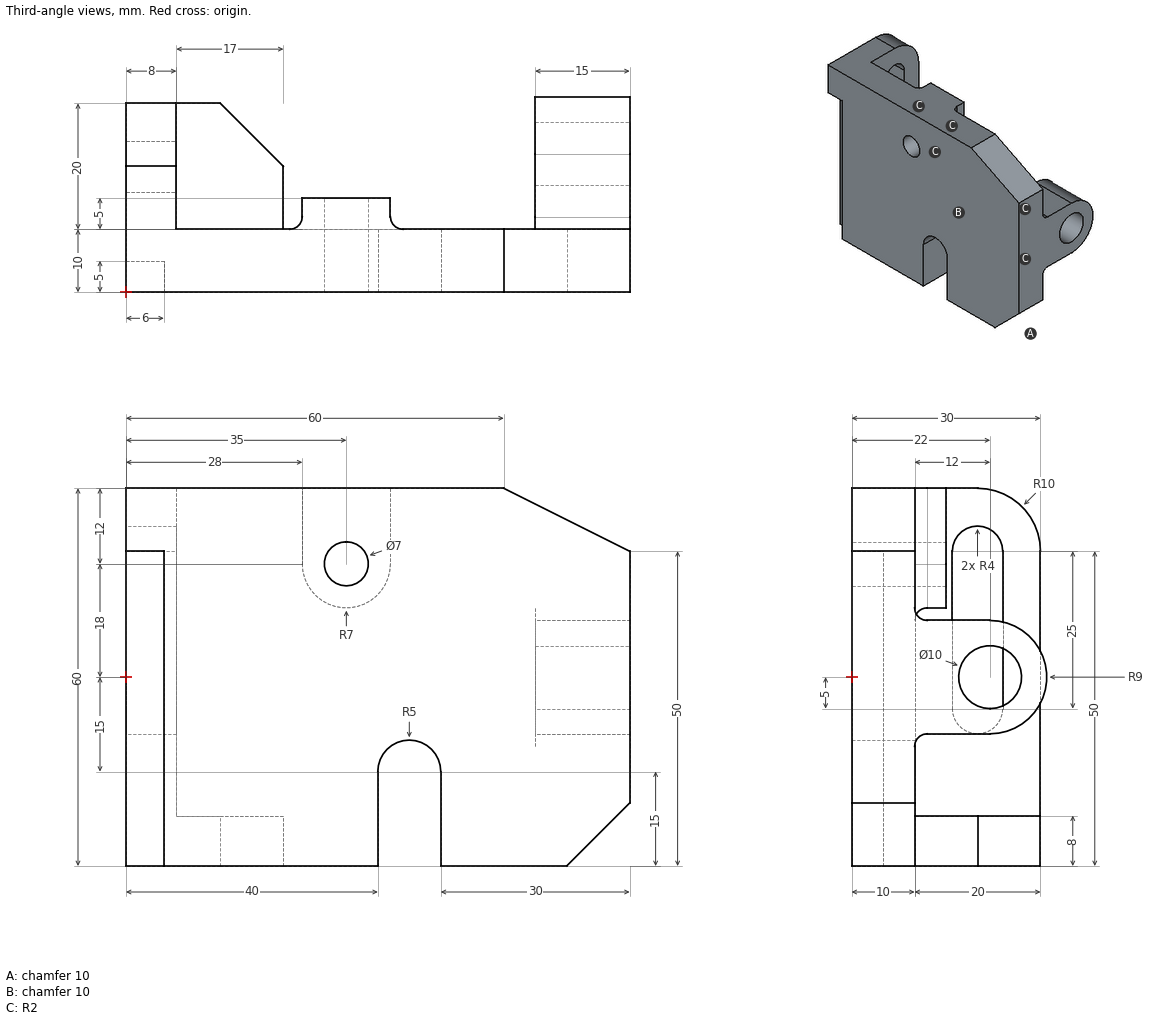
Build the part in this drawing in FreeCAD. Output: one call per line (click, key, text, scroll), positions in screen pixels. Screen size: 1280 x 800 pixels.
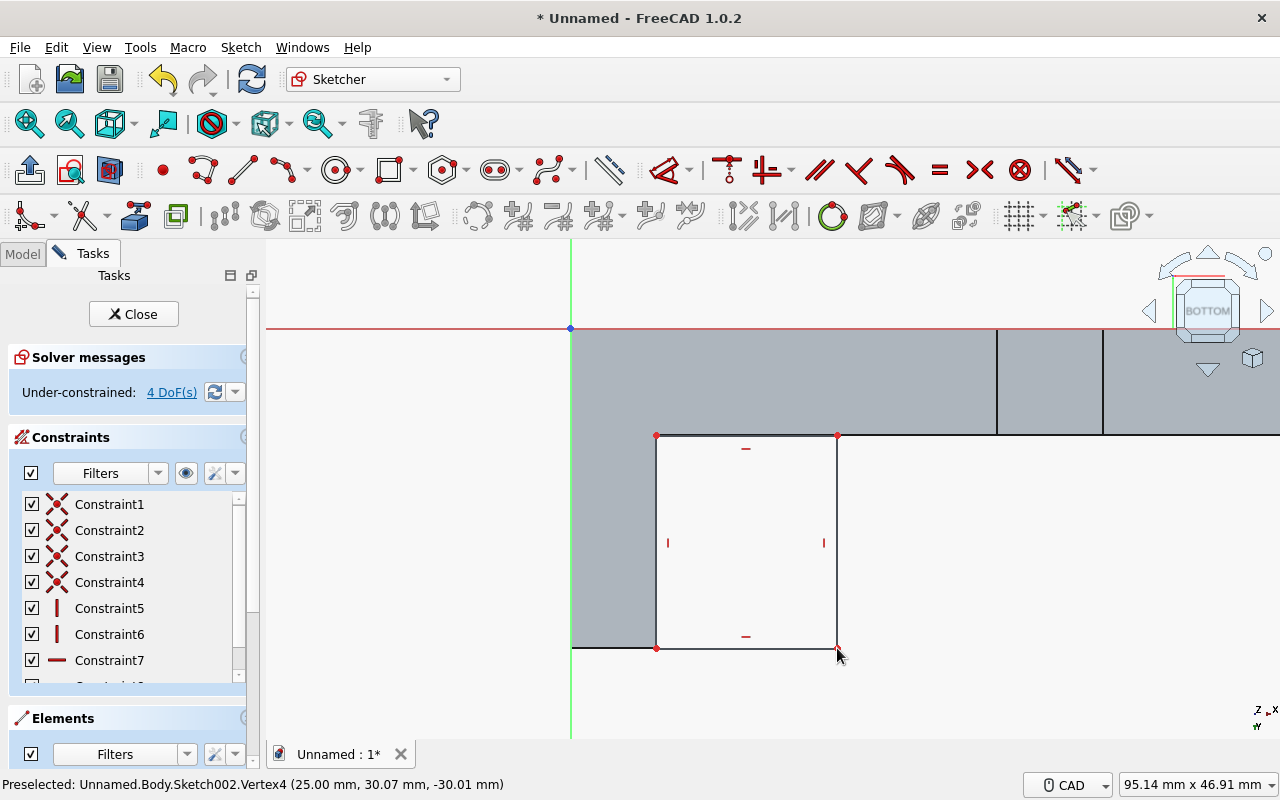
click(664, 170)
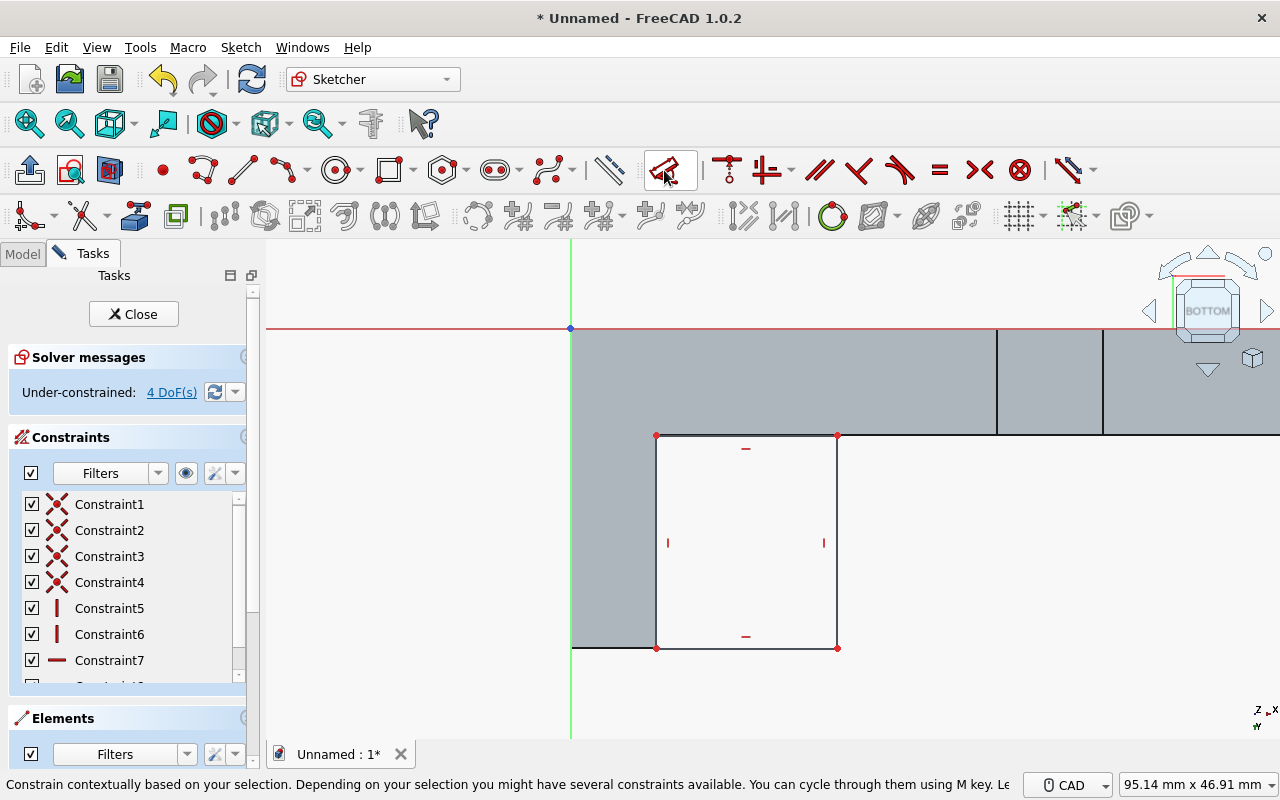
click(656, 500)
click(622, 543)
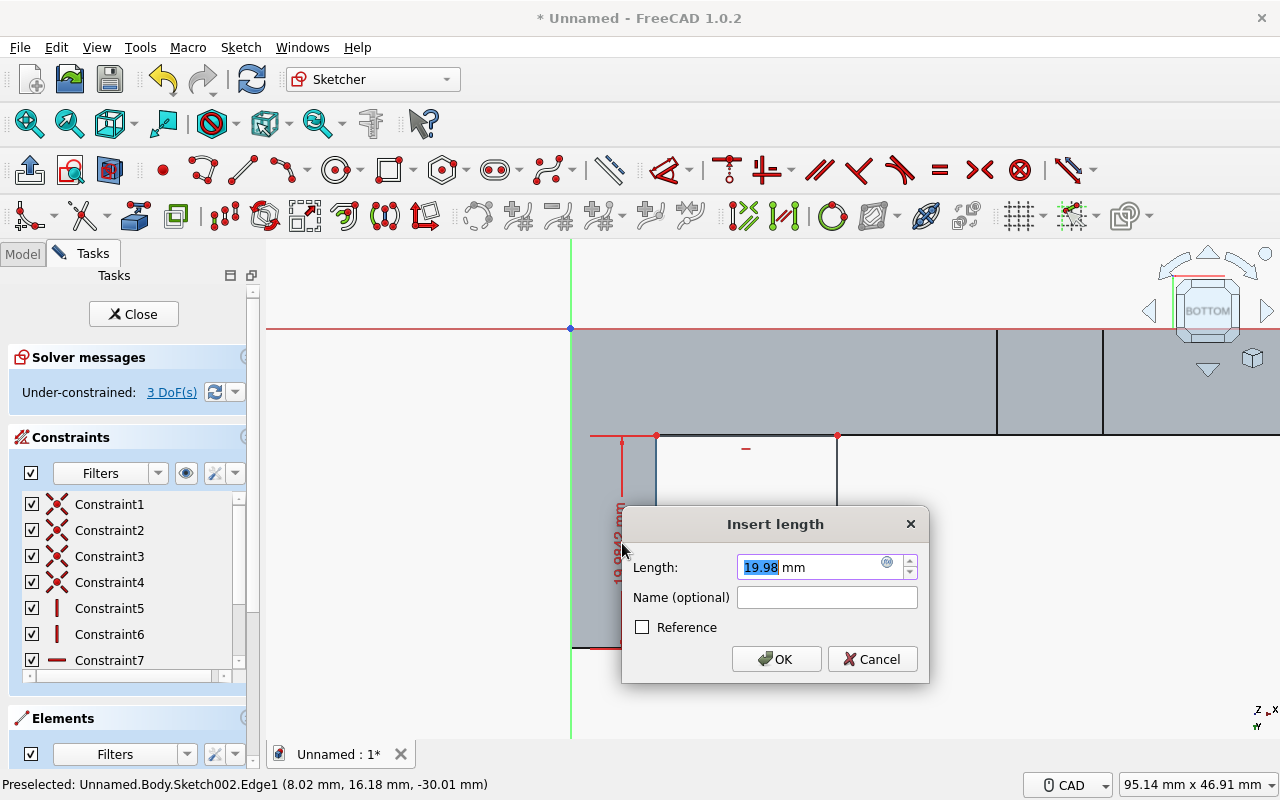
text(20)
key(Return)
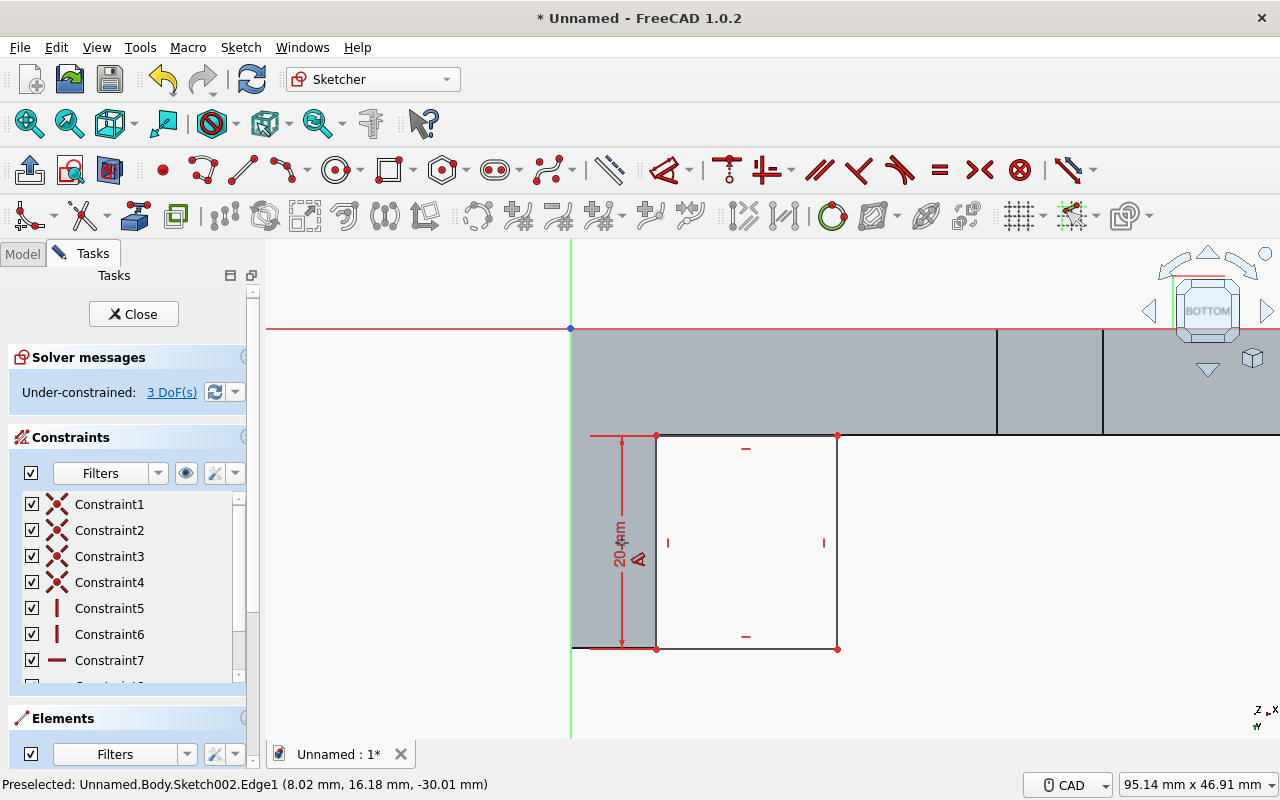
click(710, 649)
click(747, 683)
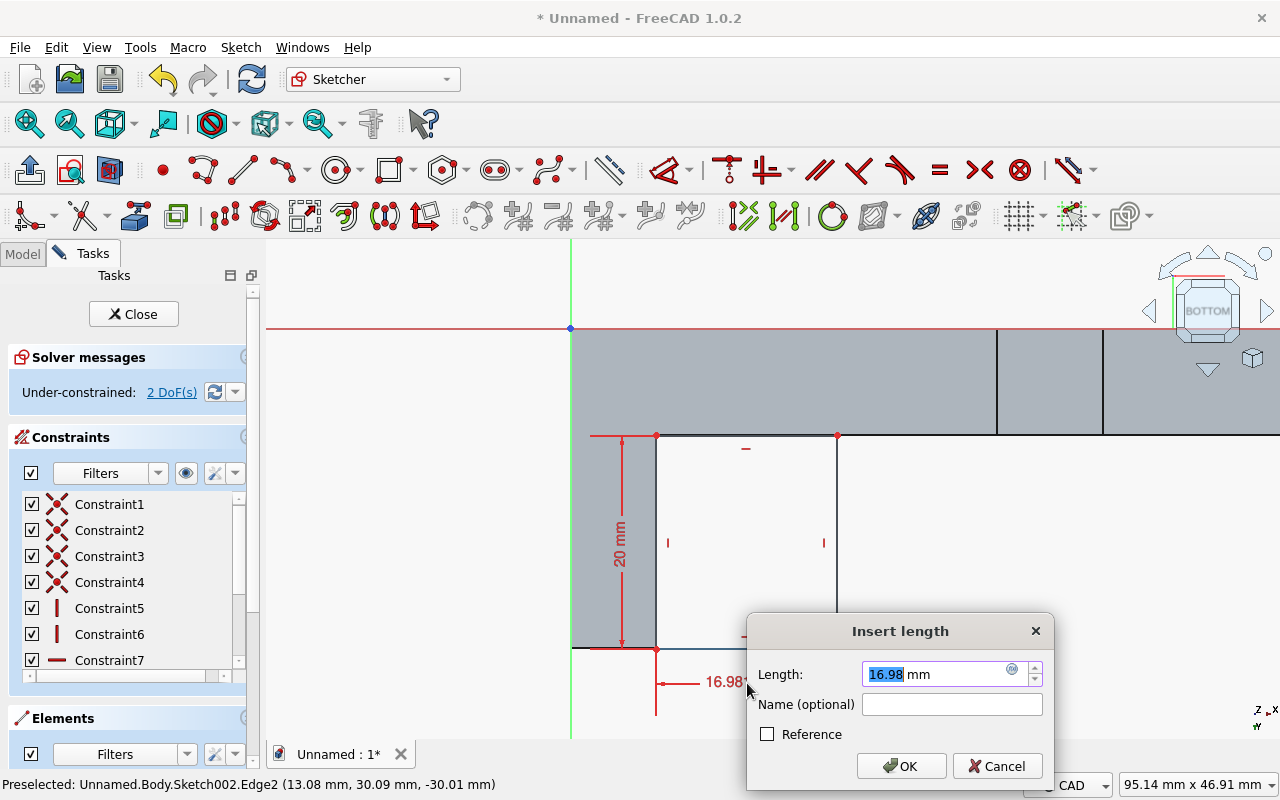
text(17)
key(Return)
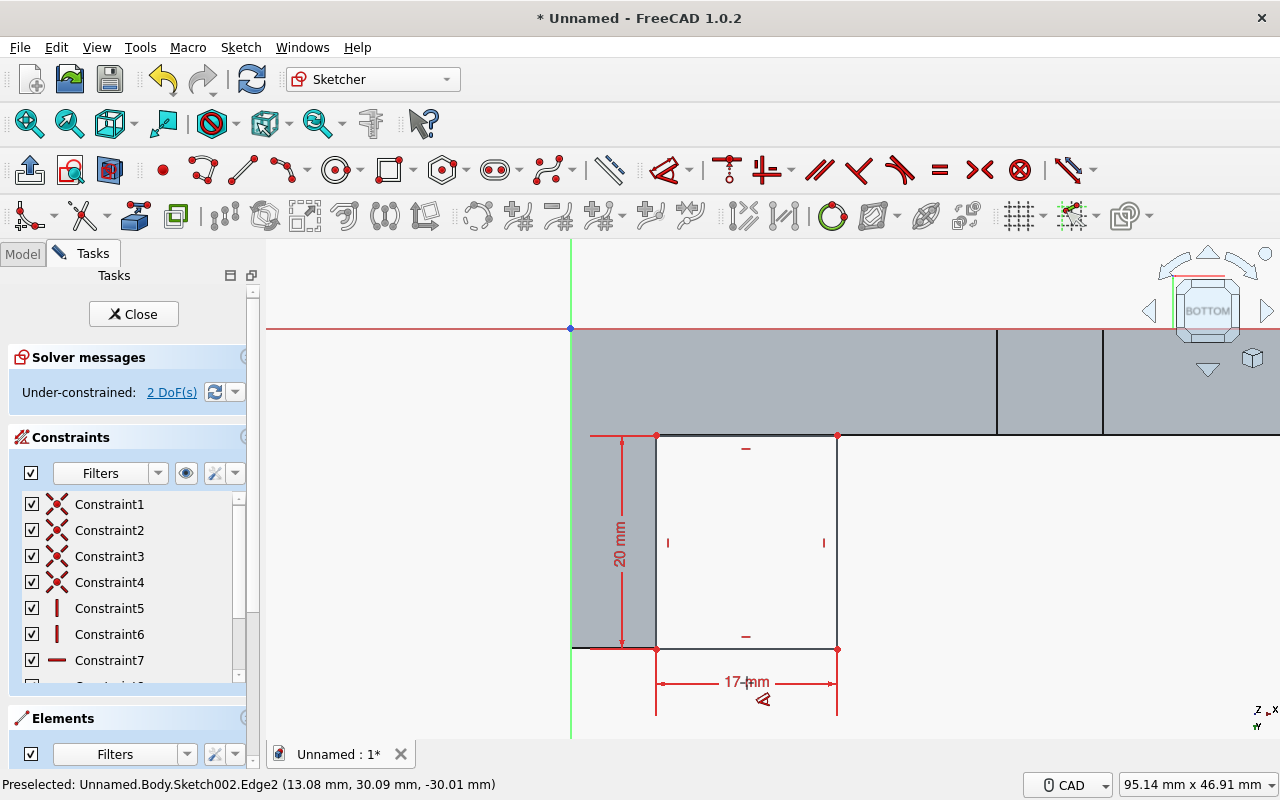
click(656, 436)
click(613, 295)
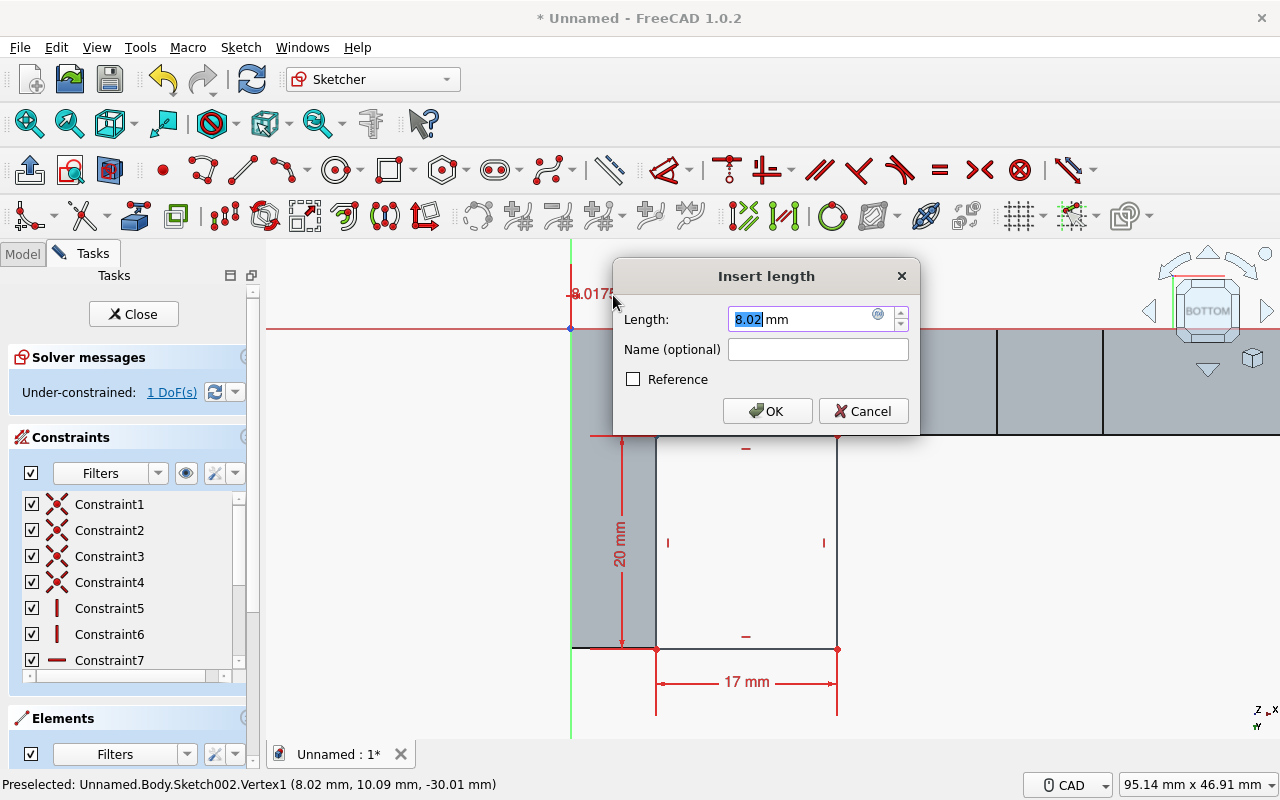
text(8)
key(Return)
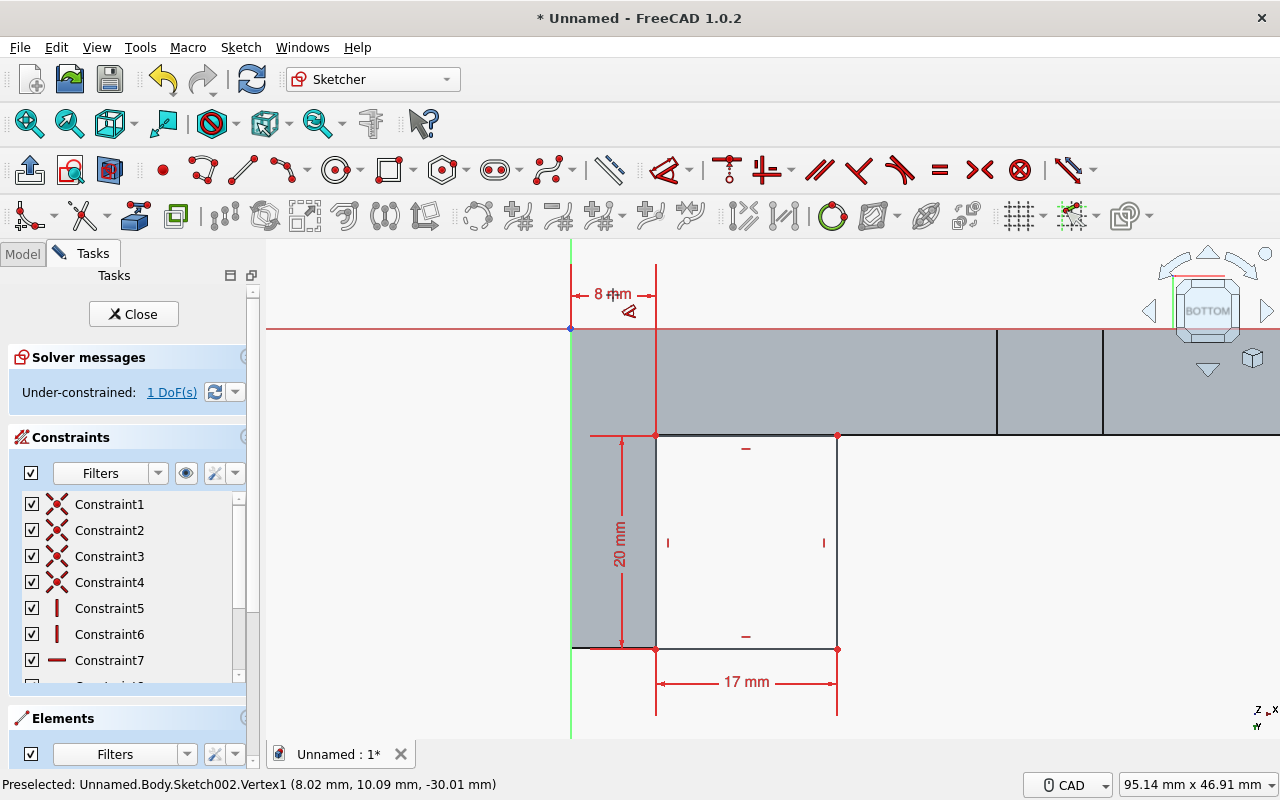
click(656, 436)
click(537, 382)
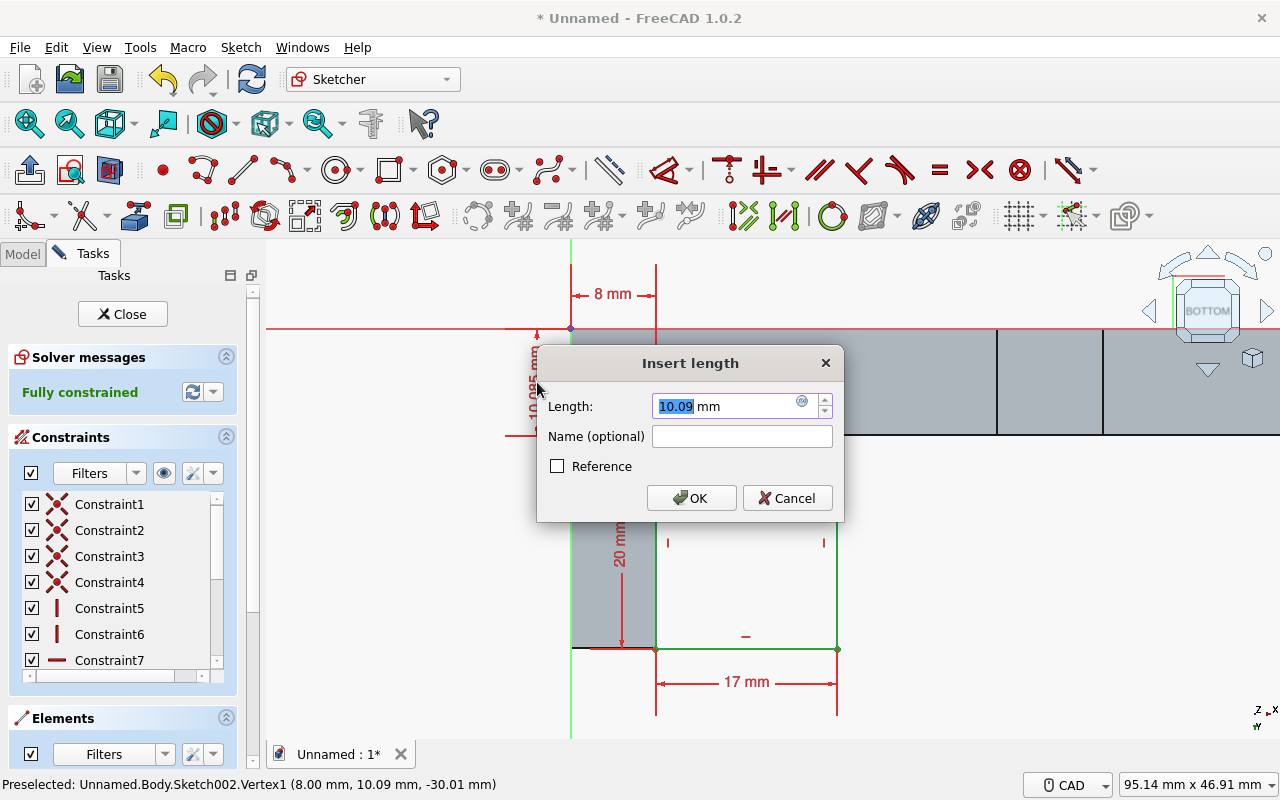
text(10)
key(Return)
key(Escape)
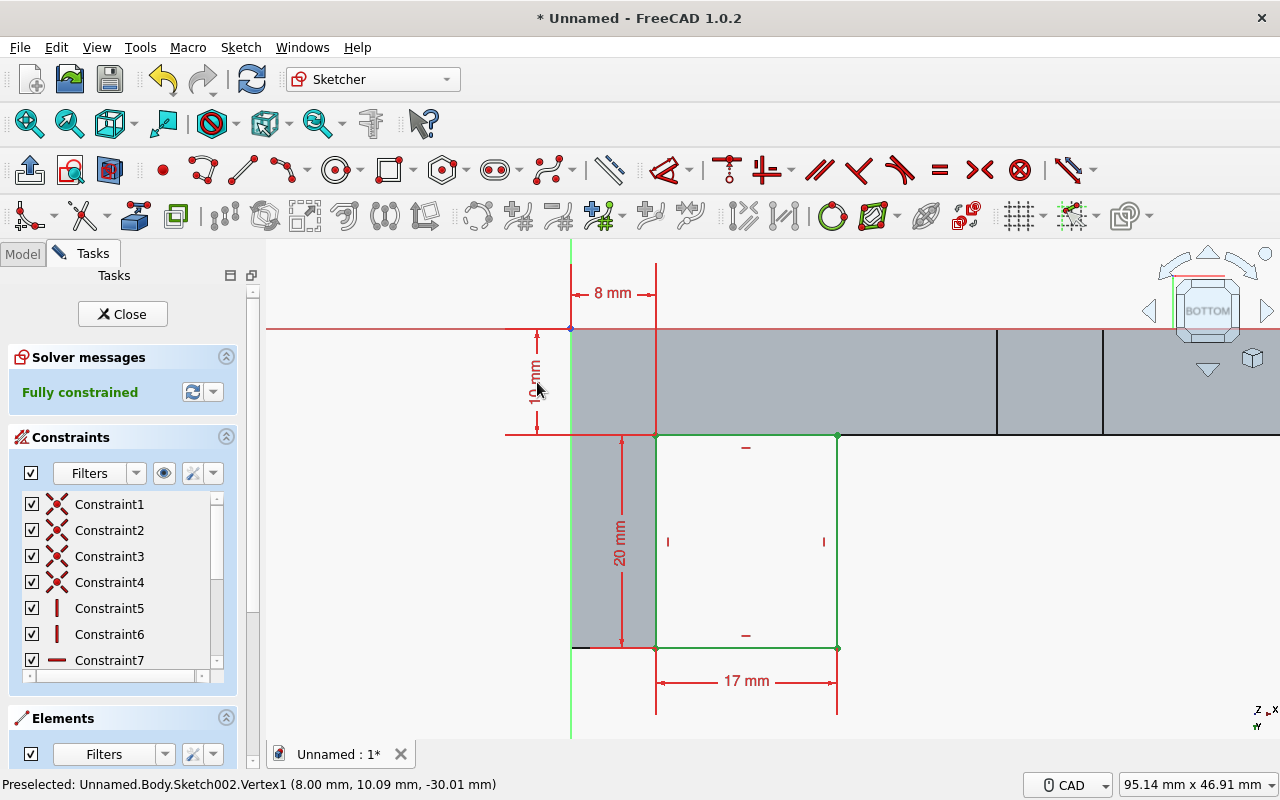
click(123, 314)